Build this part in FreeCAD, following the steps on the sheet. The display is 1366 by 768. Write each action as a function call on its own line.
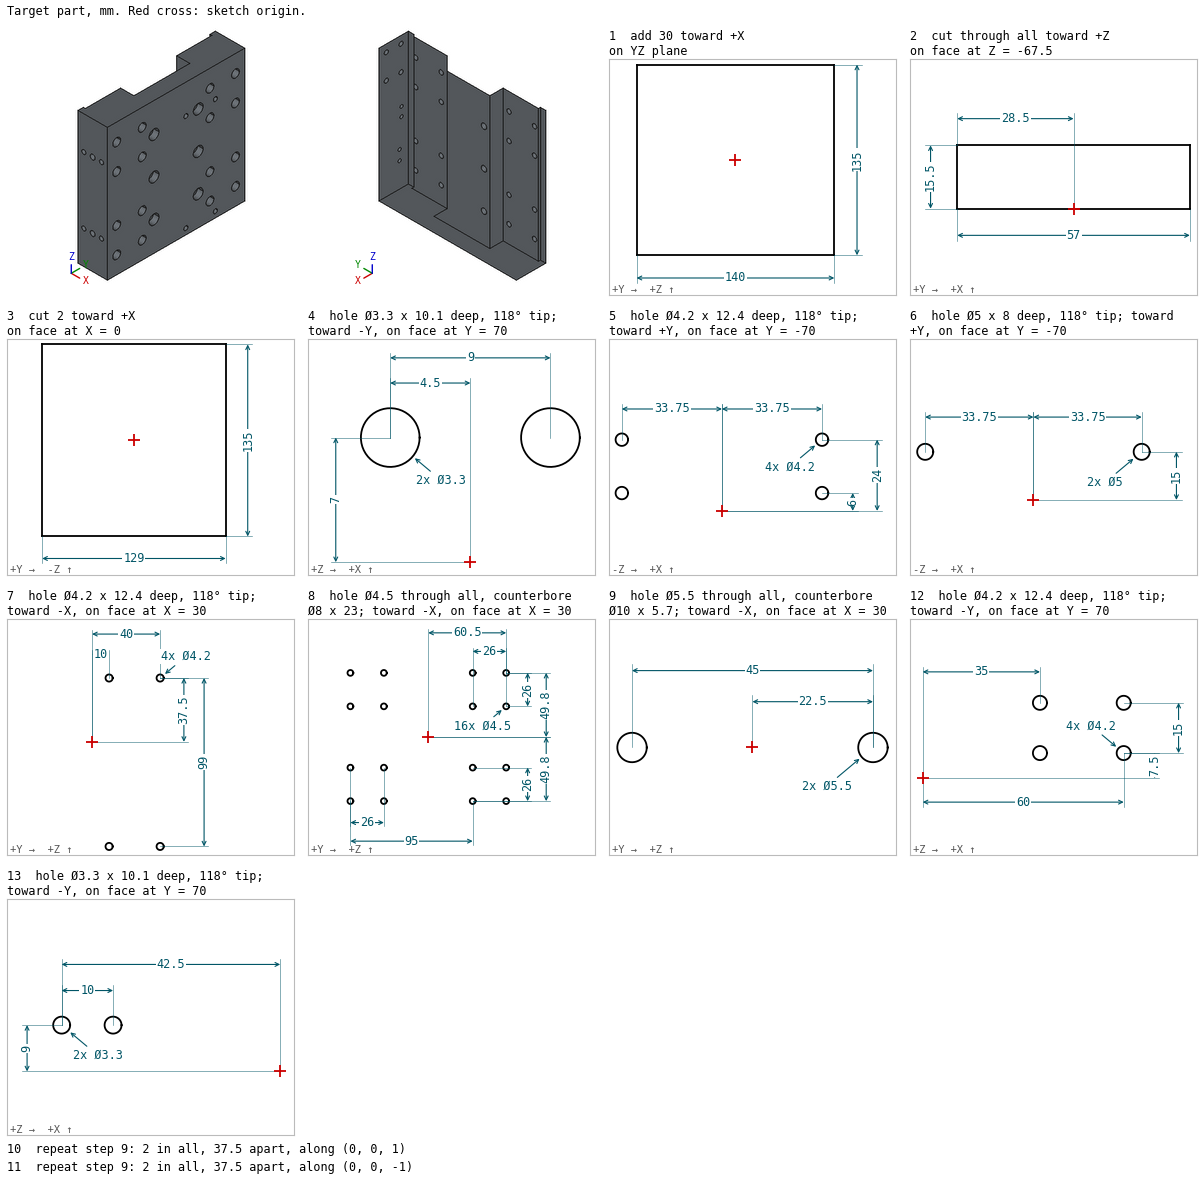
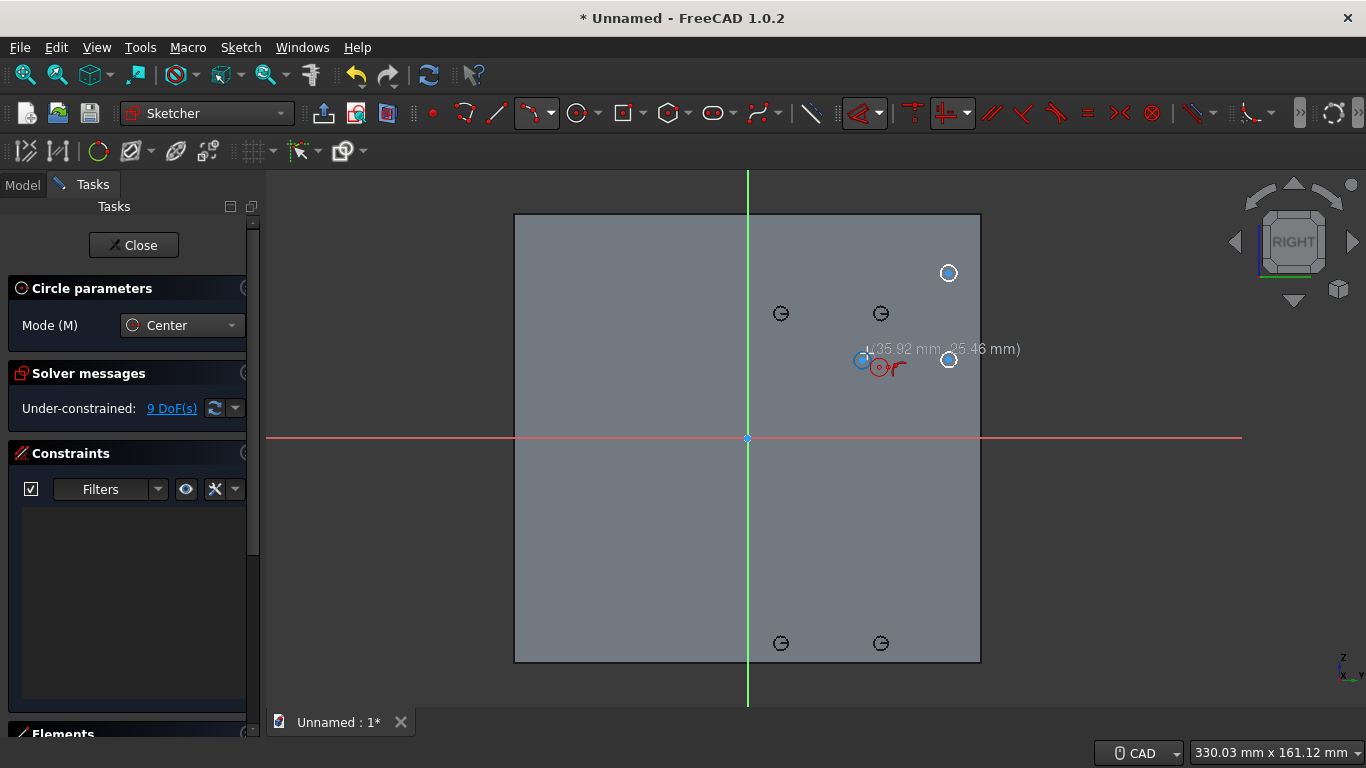
scroll(863, 273, up, 6)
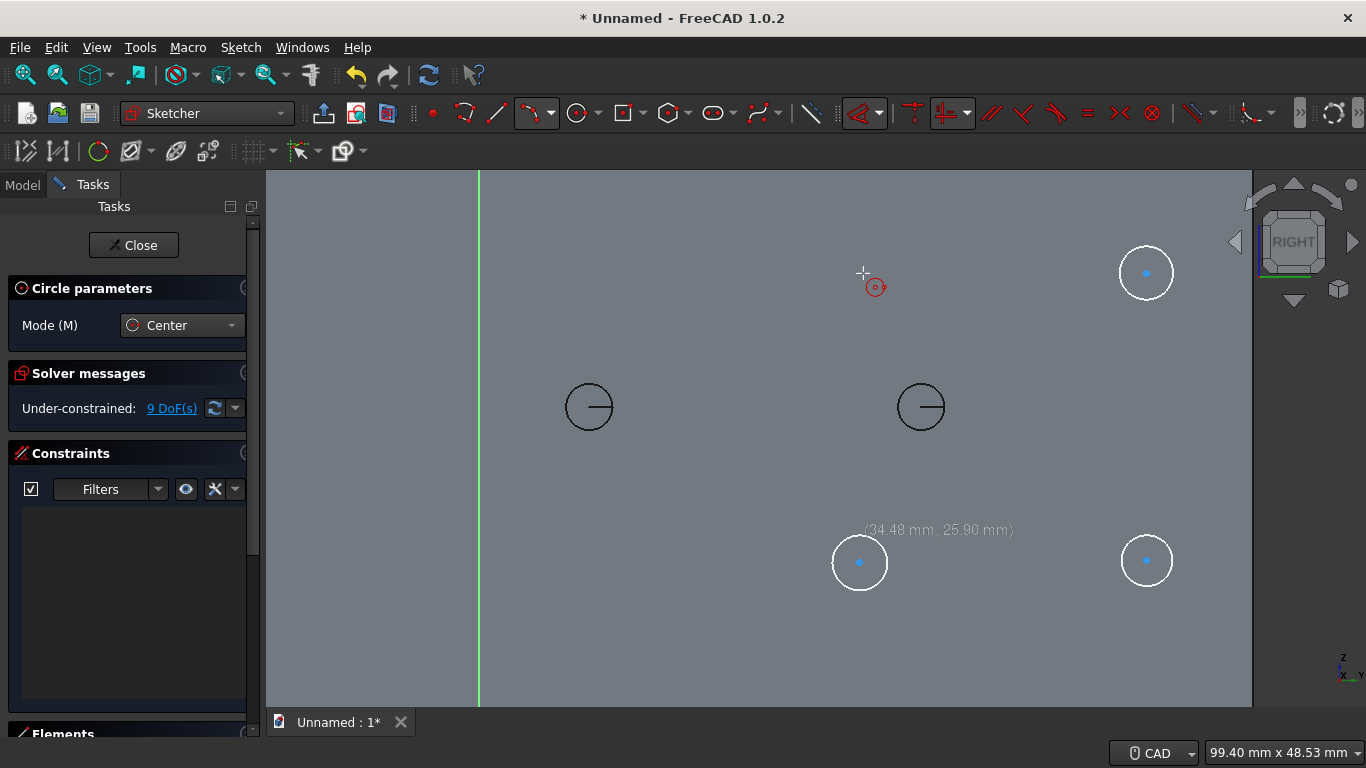
scroll(863, 273, down, 6)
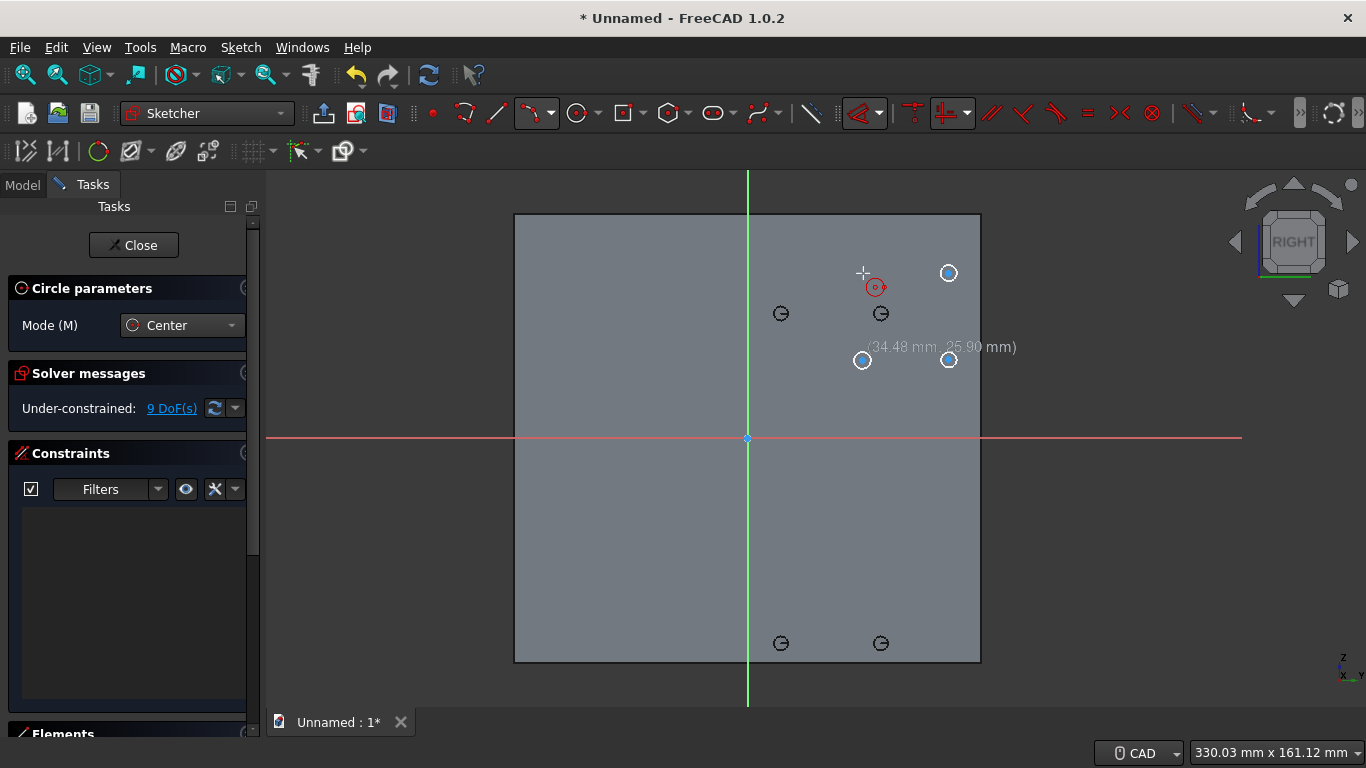
click(863, 273)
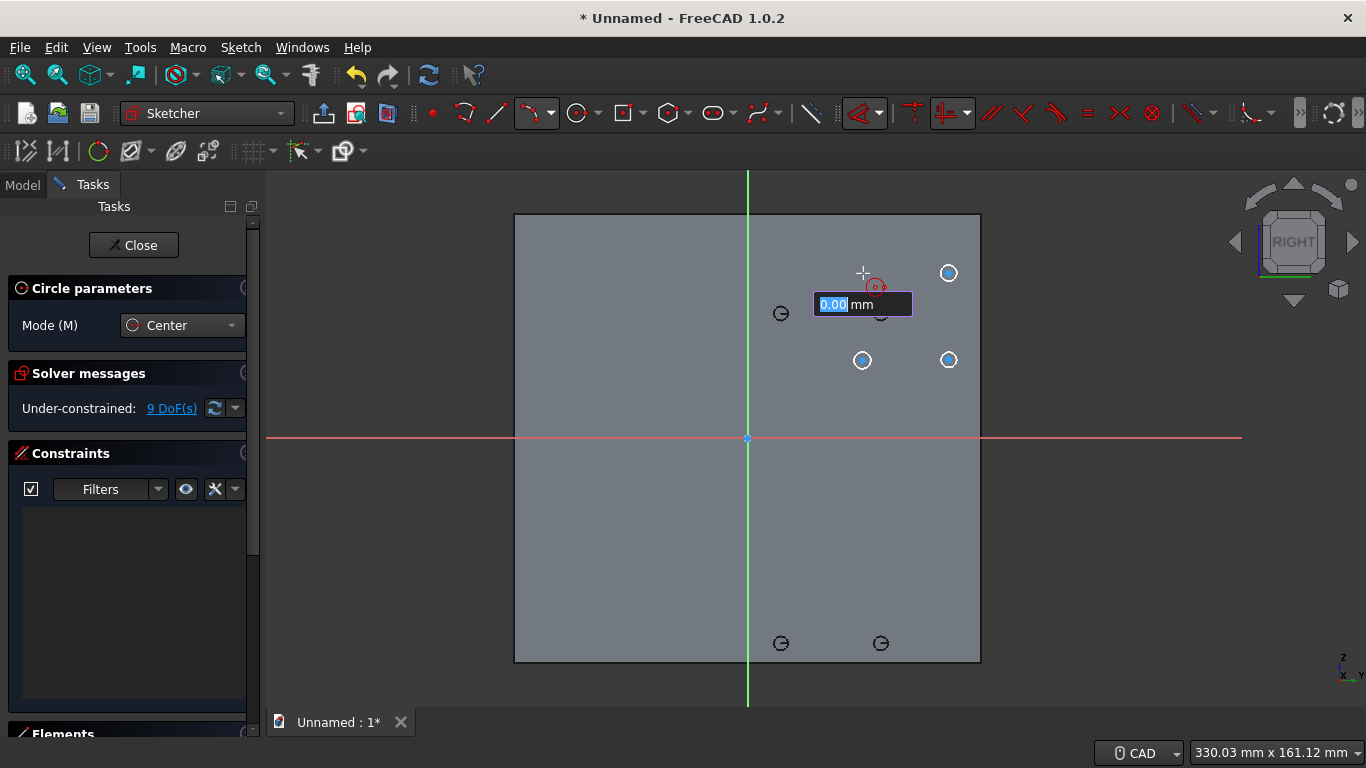
scroll(868, 267, up, 4)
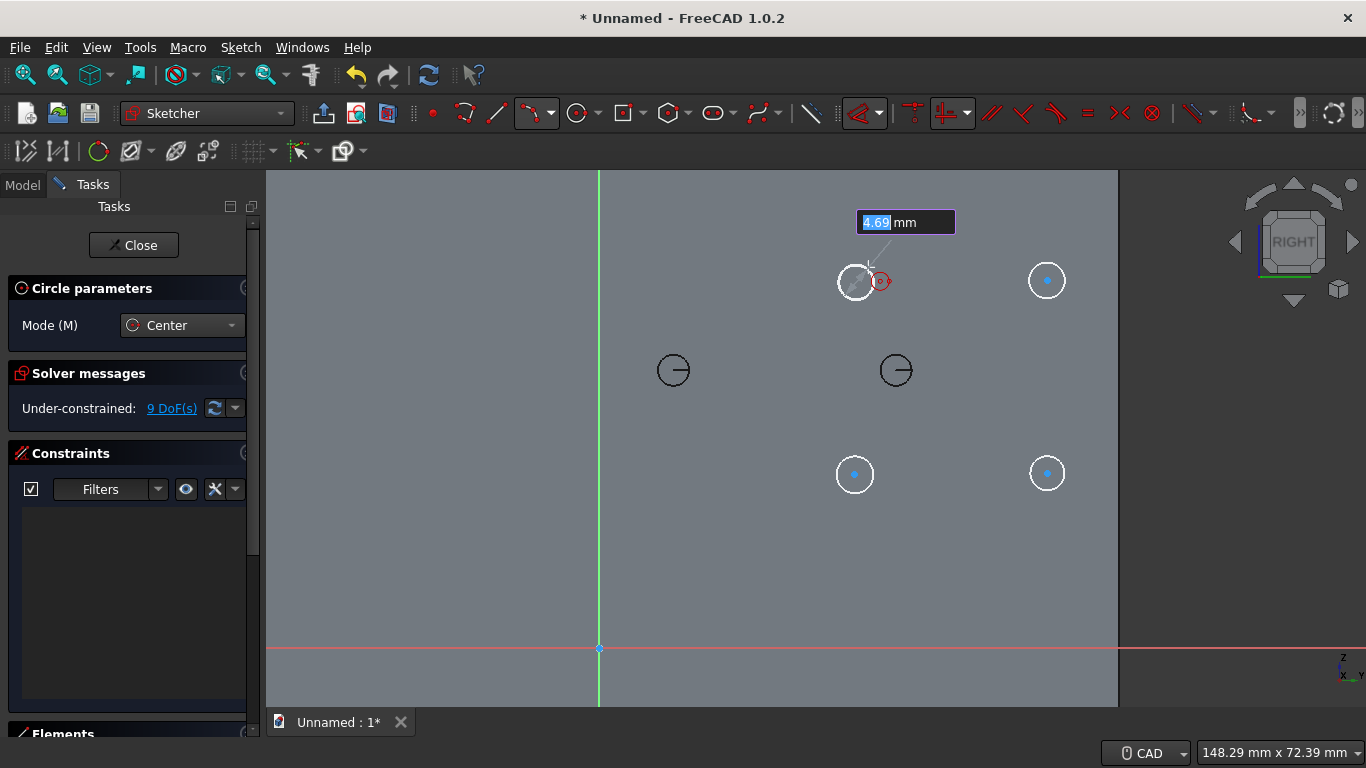
click(867, 267)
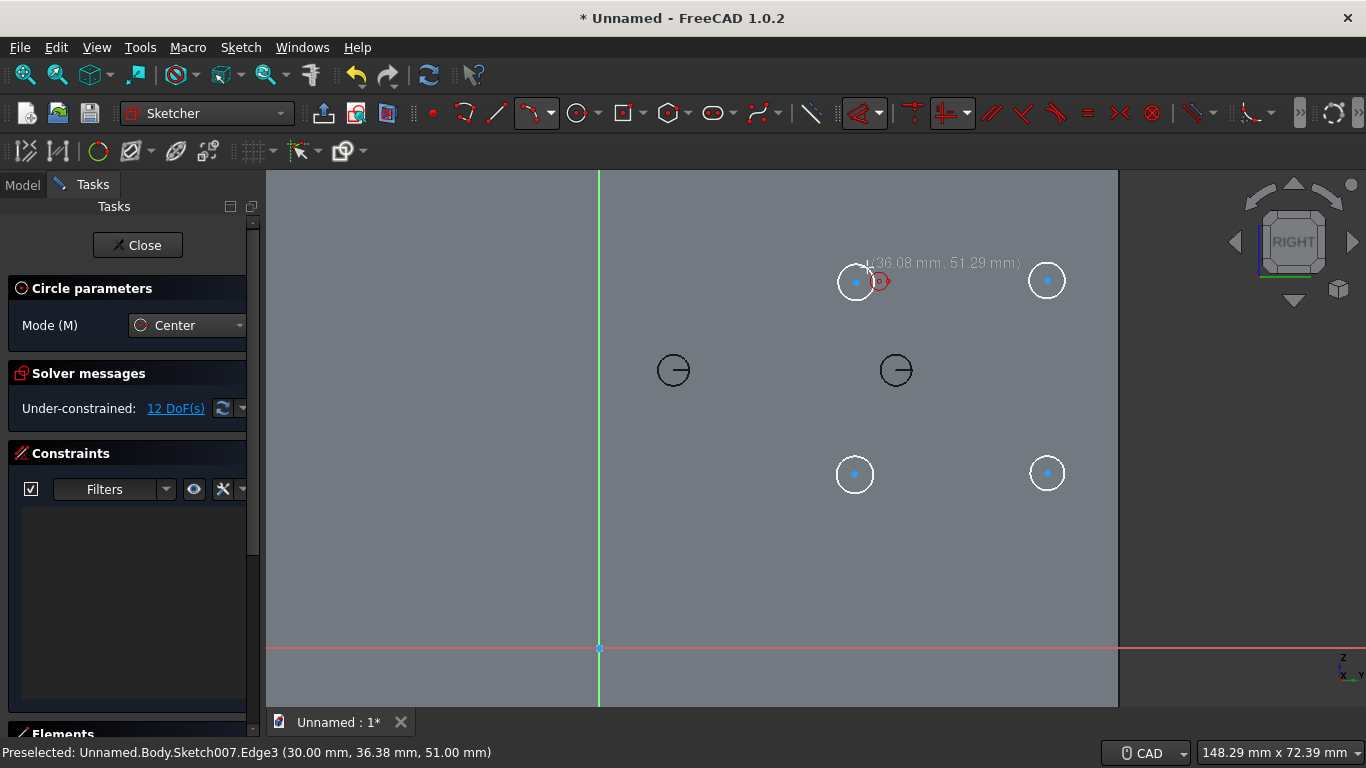
scroll(868, 267, down, 4)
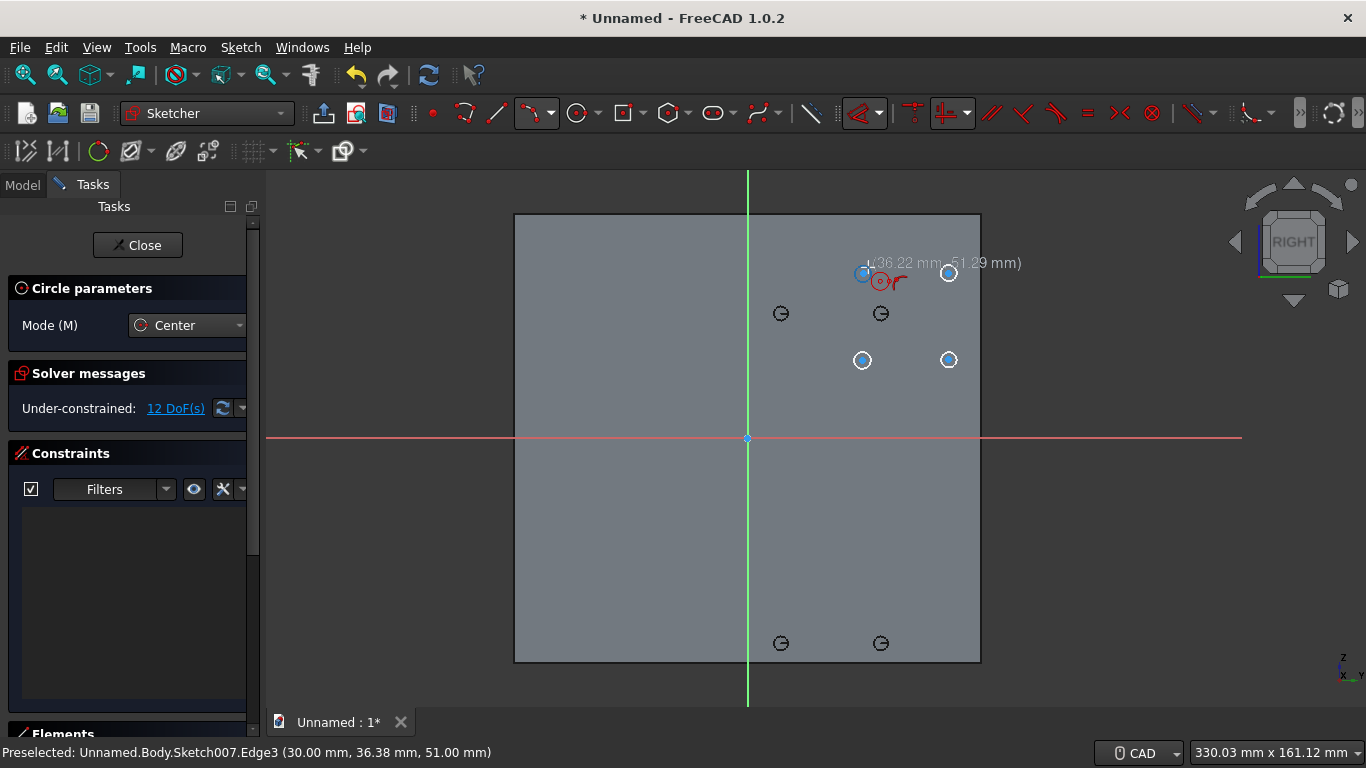
scroll(863, 604, up, 6)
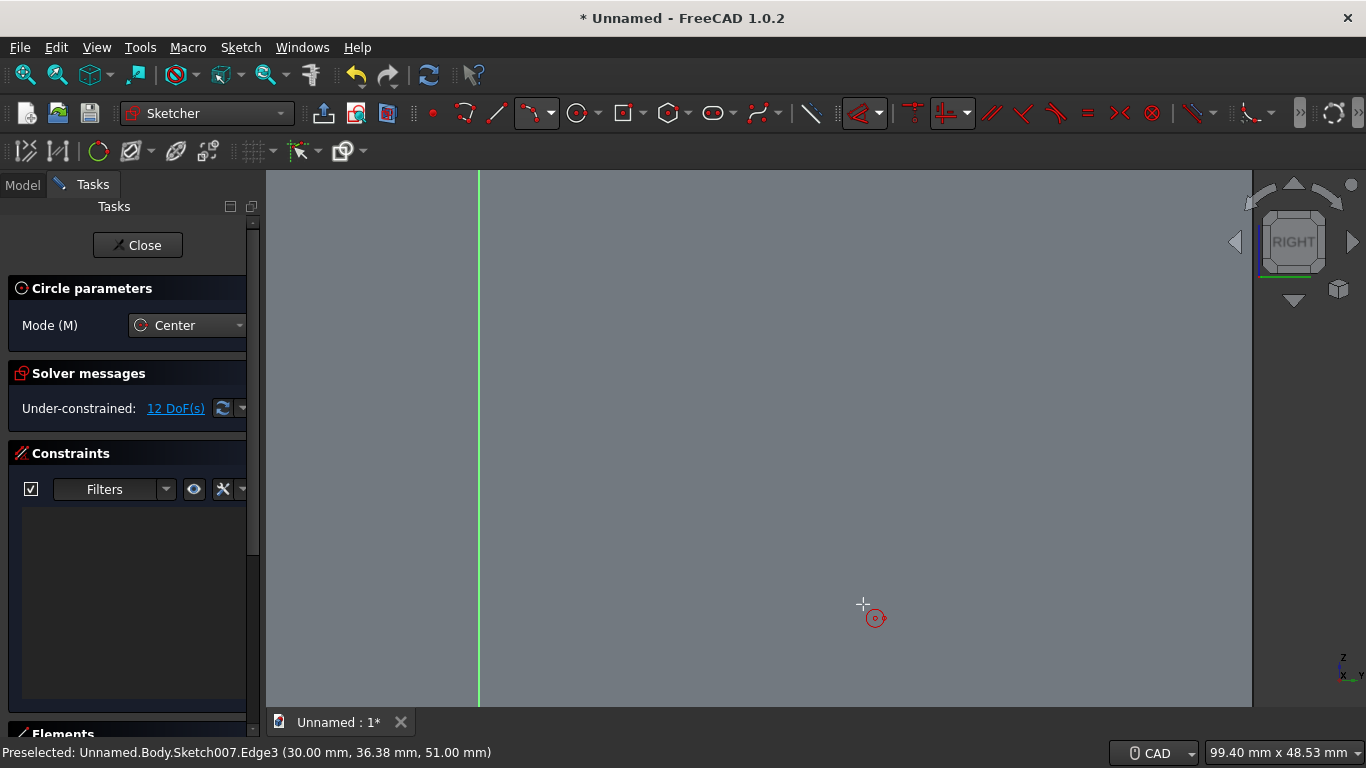
scroll(863, 605, down, 6)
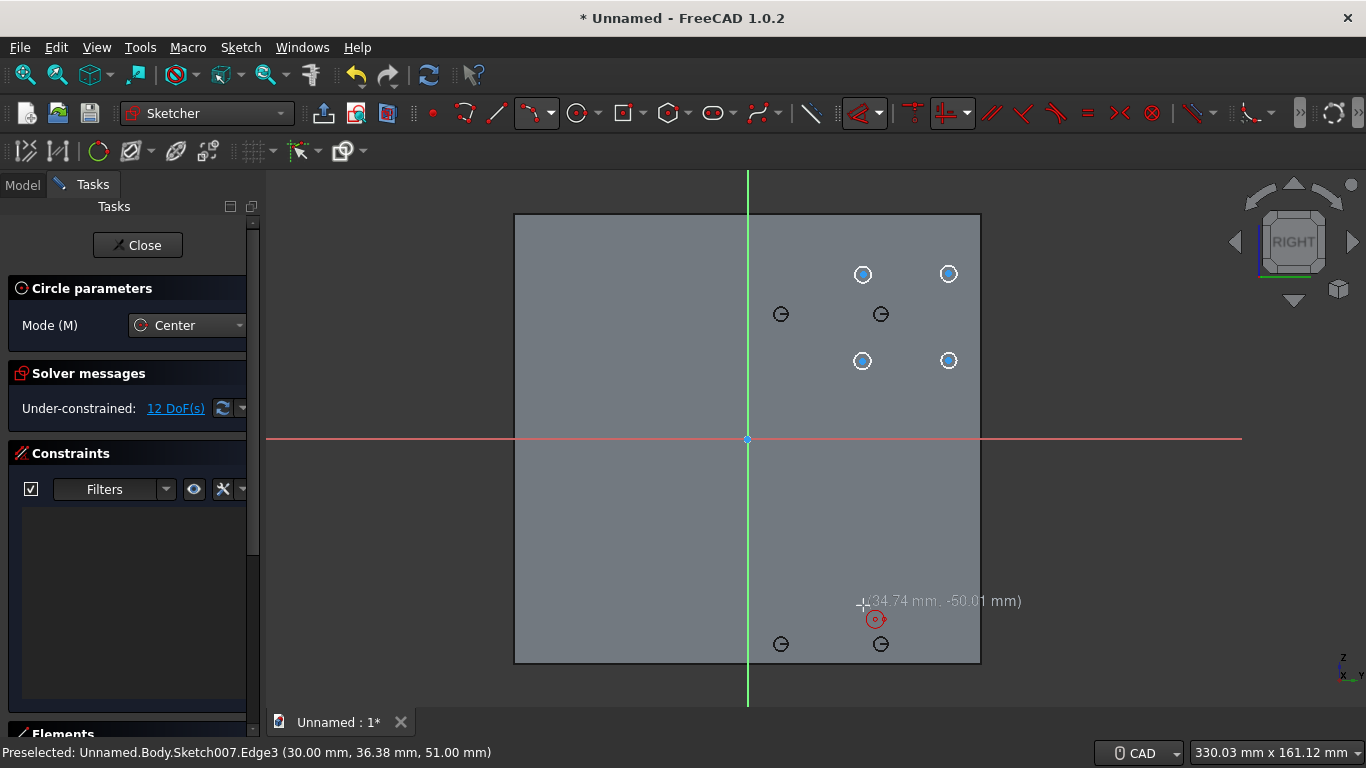
click(863, 605)